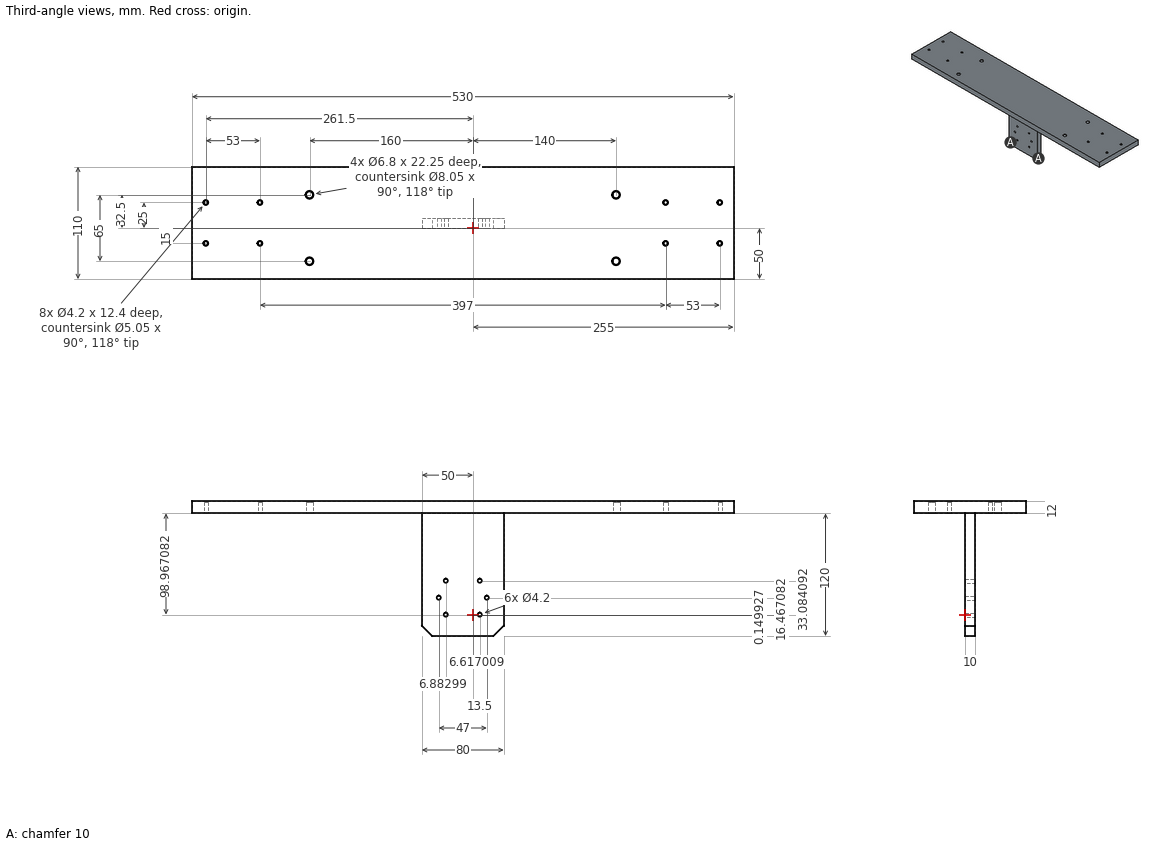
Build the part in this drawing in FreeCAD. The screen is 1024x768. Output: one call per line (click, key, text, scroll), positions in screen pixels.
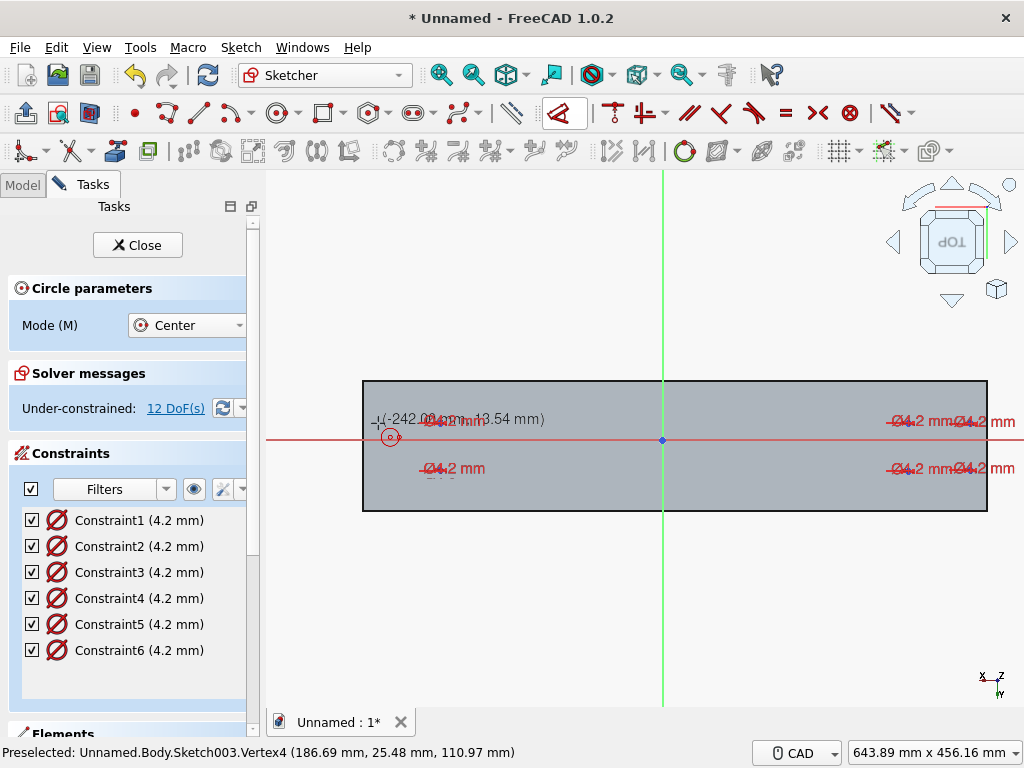
click(379, 423)
move(380, 421)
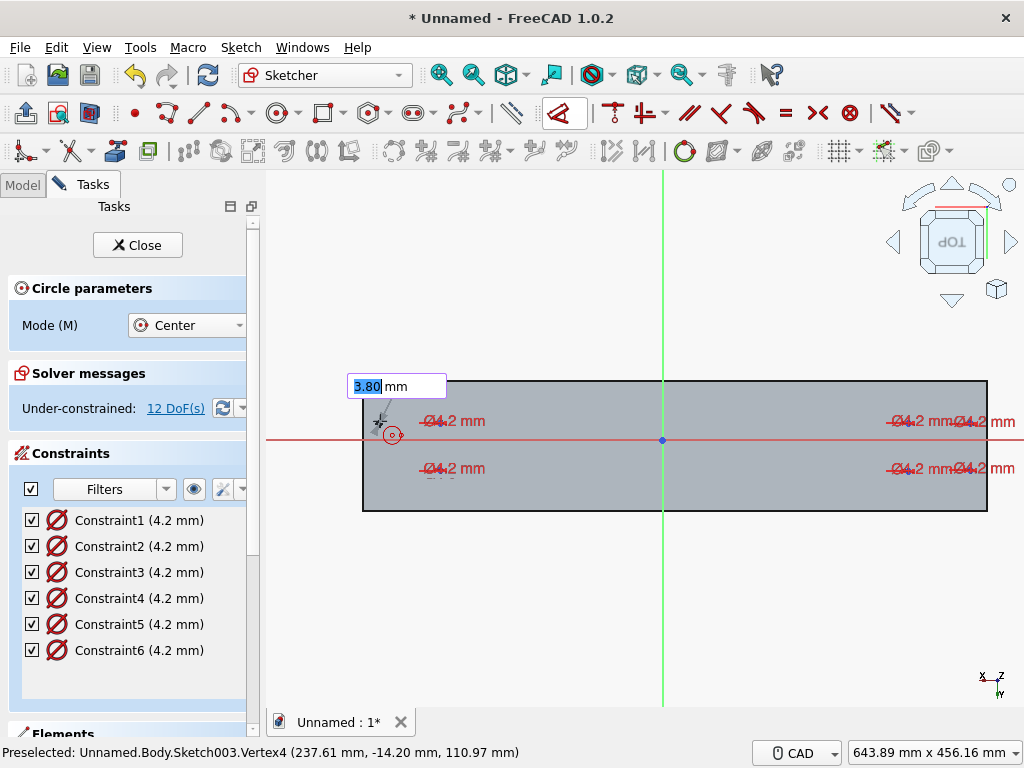
text(4.2)
key(Return)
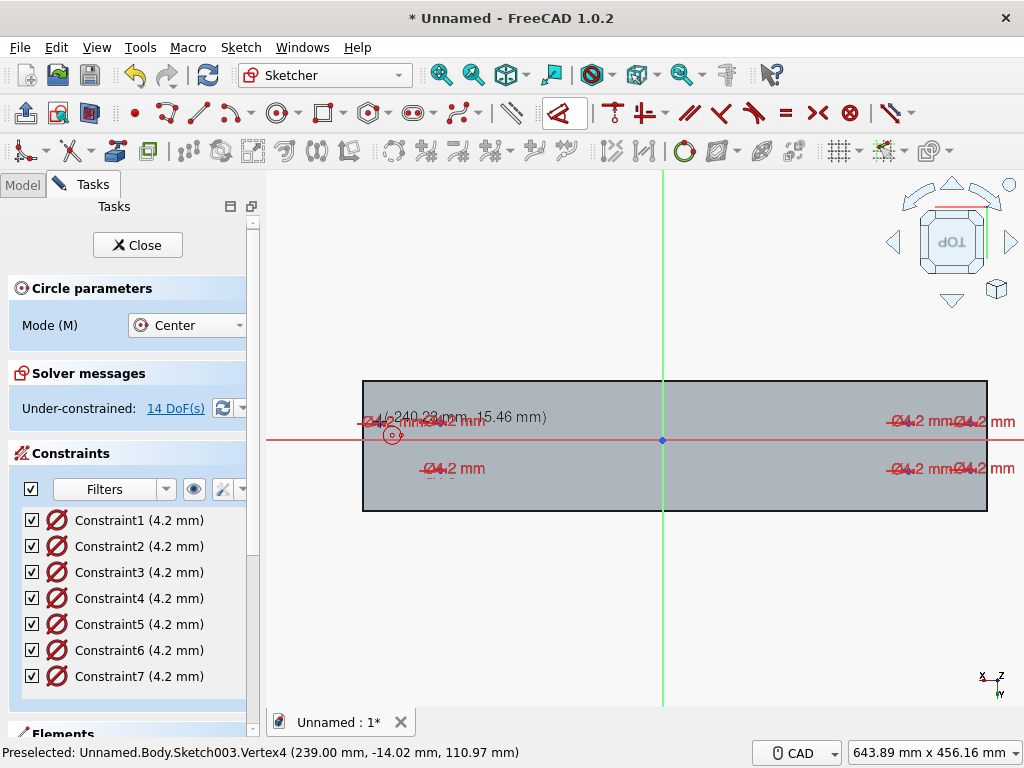
scroll(379, 470, up, 12)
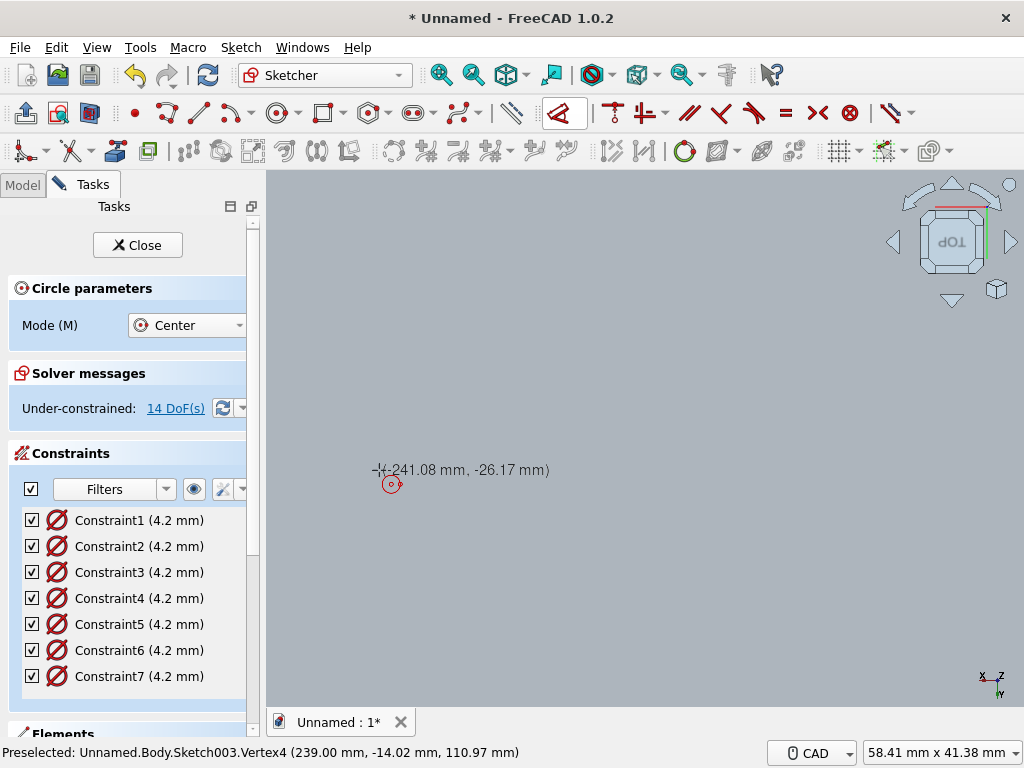
scroll(378, 454, down, 14)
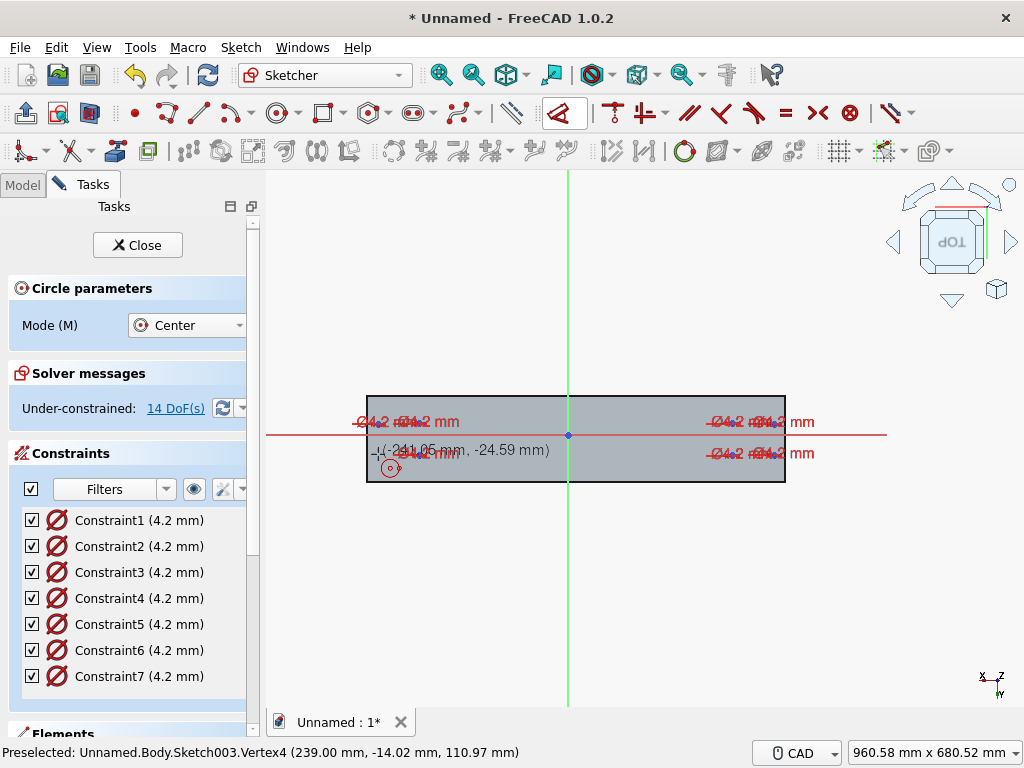
click(378, 455)
move(379, 454)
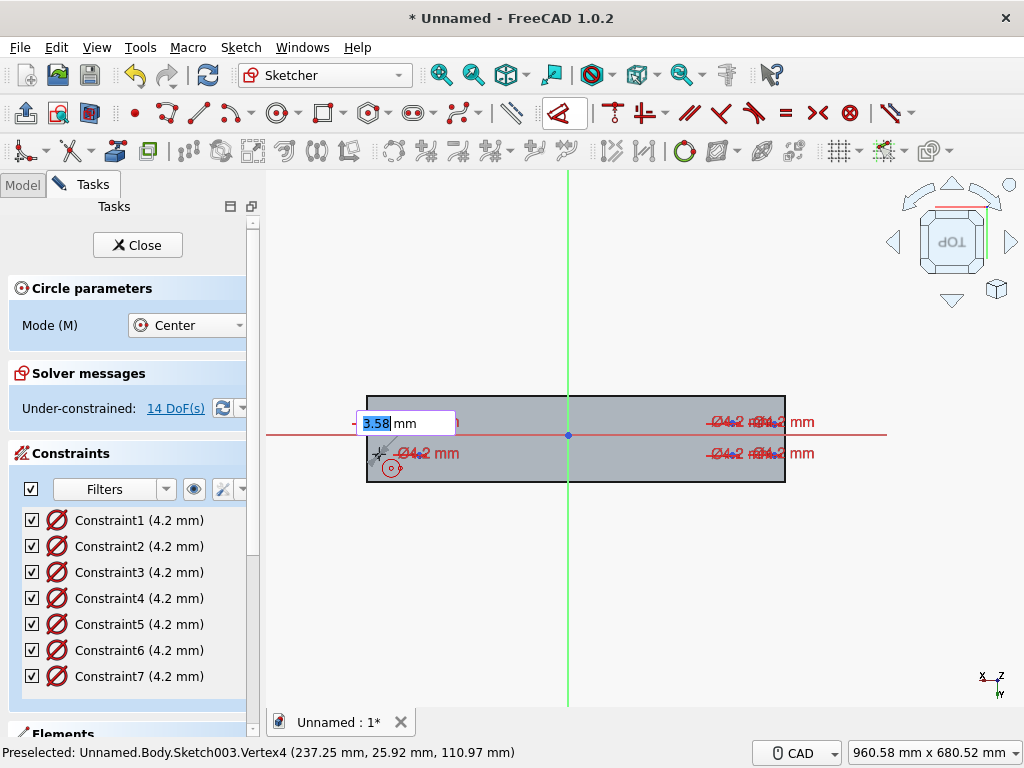
text(4.2)
key(Return)
key(Escape)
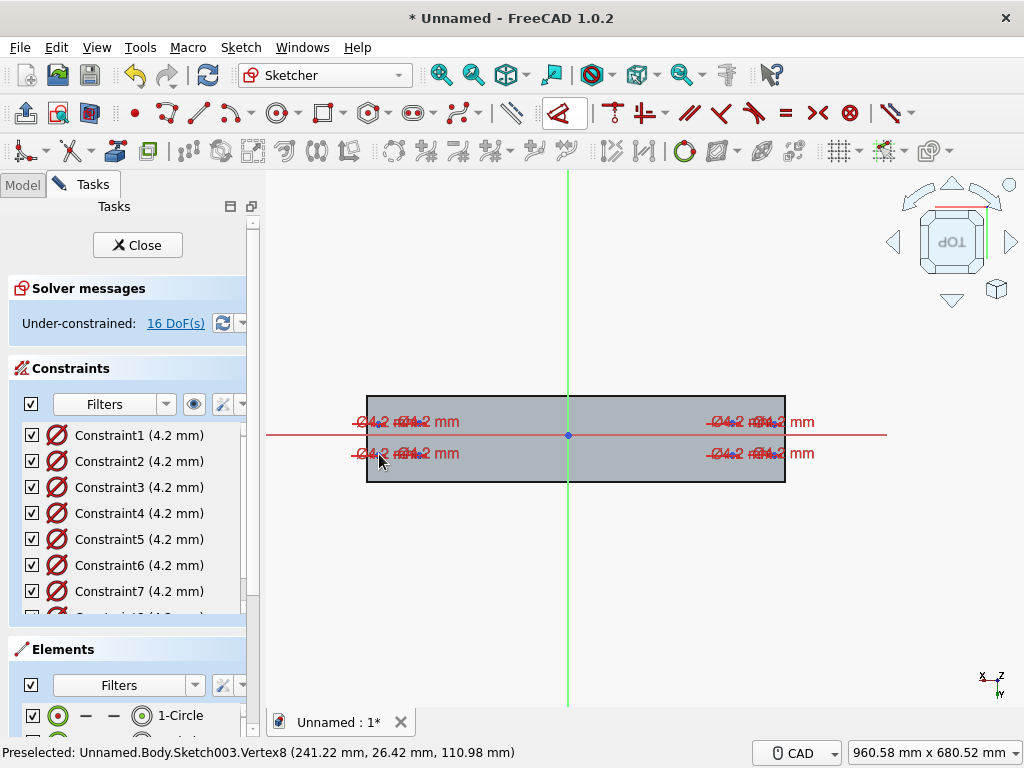
click(775, 455)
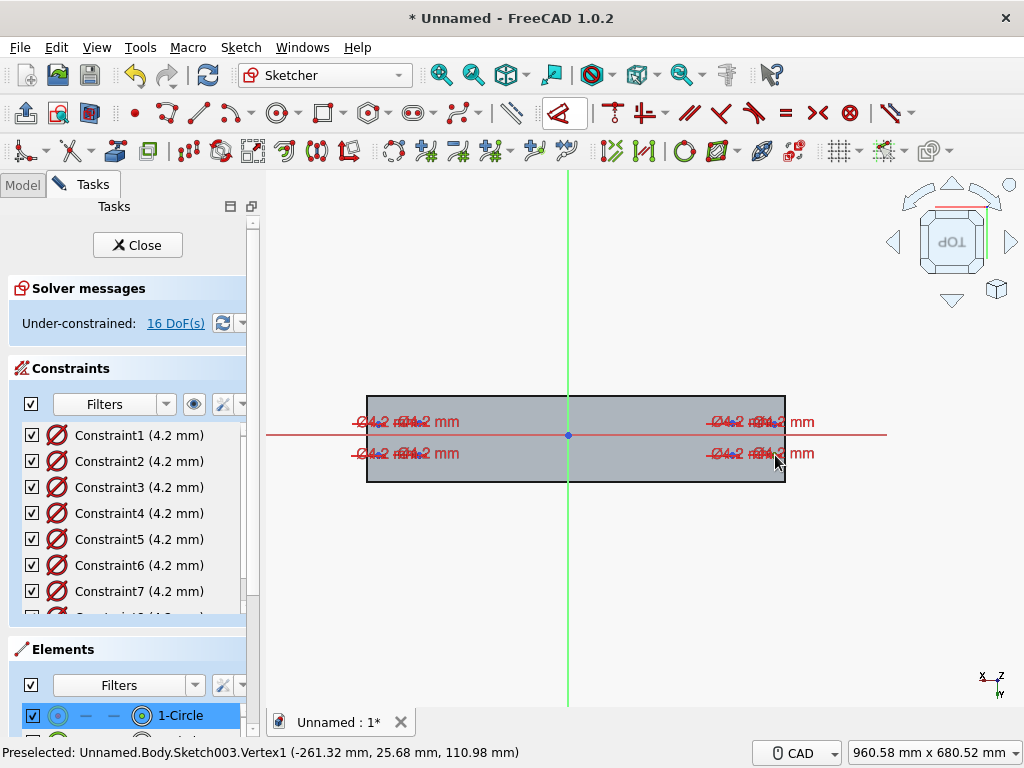
click(775, 424)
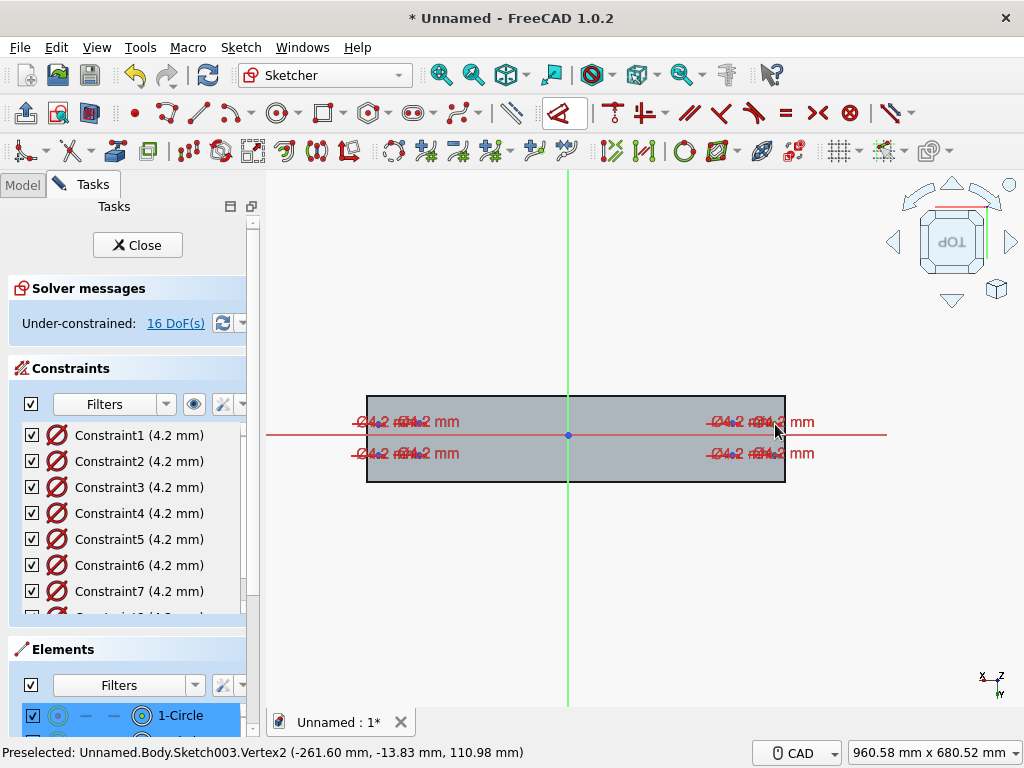
key(v)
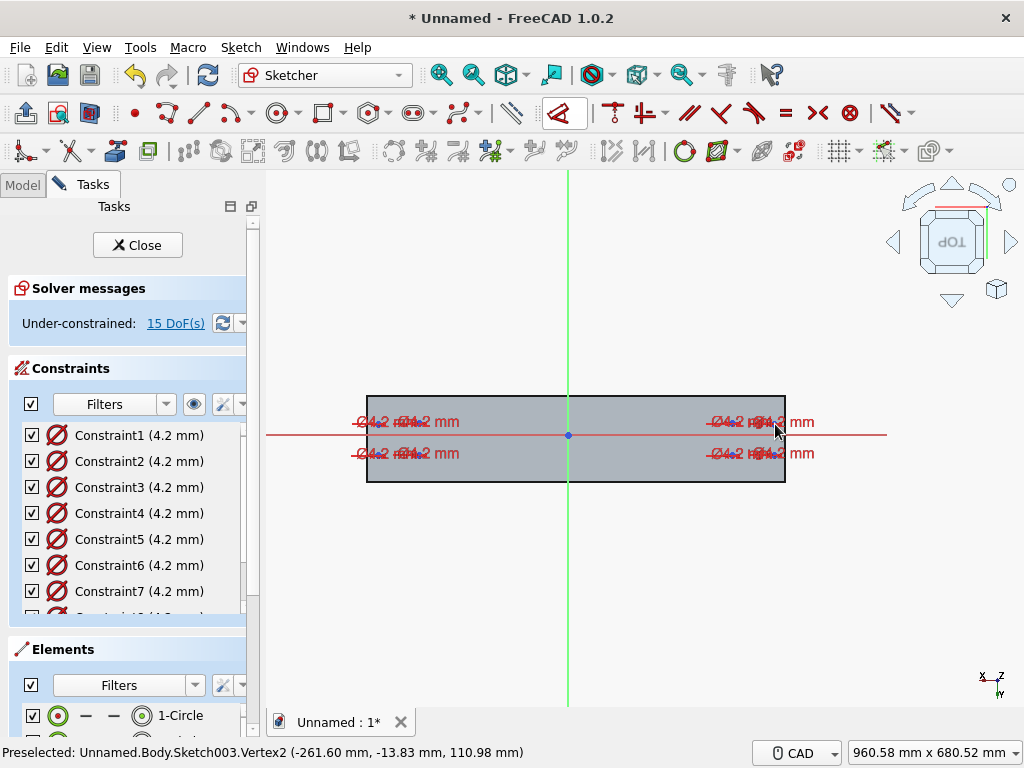
click(775, 455)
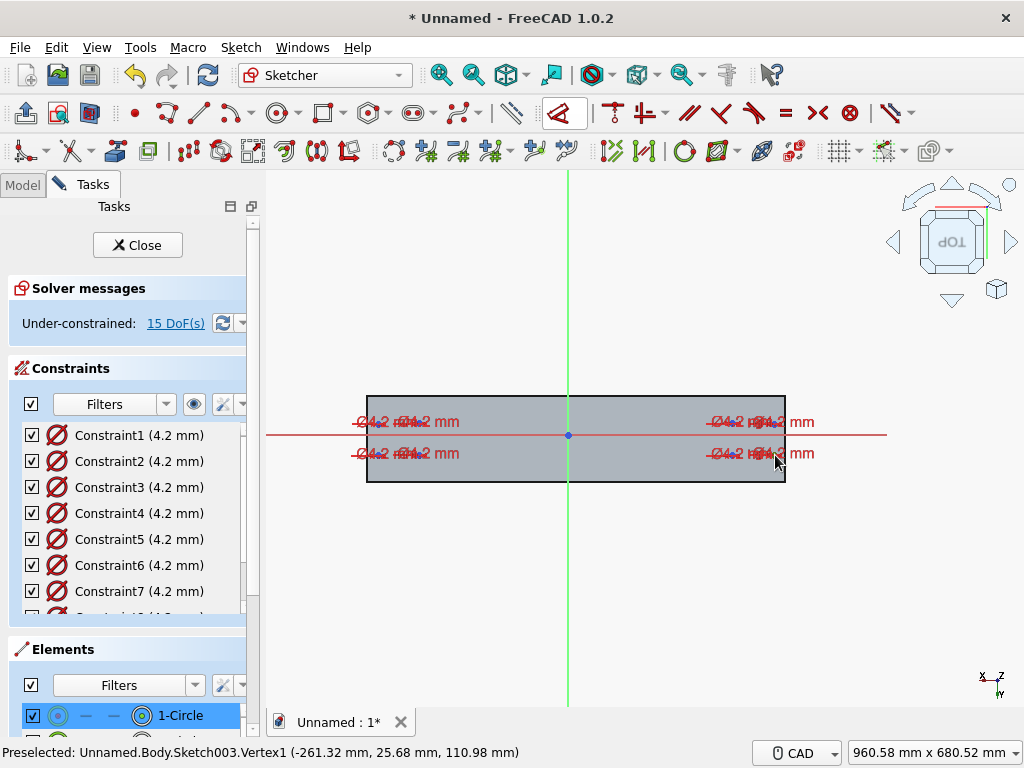
click(733, 456)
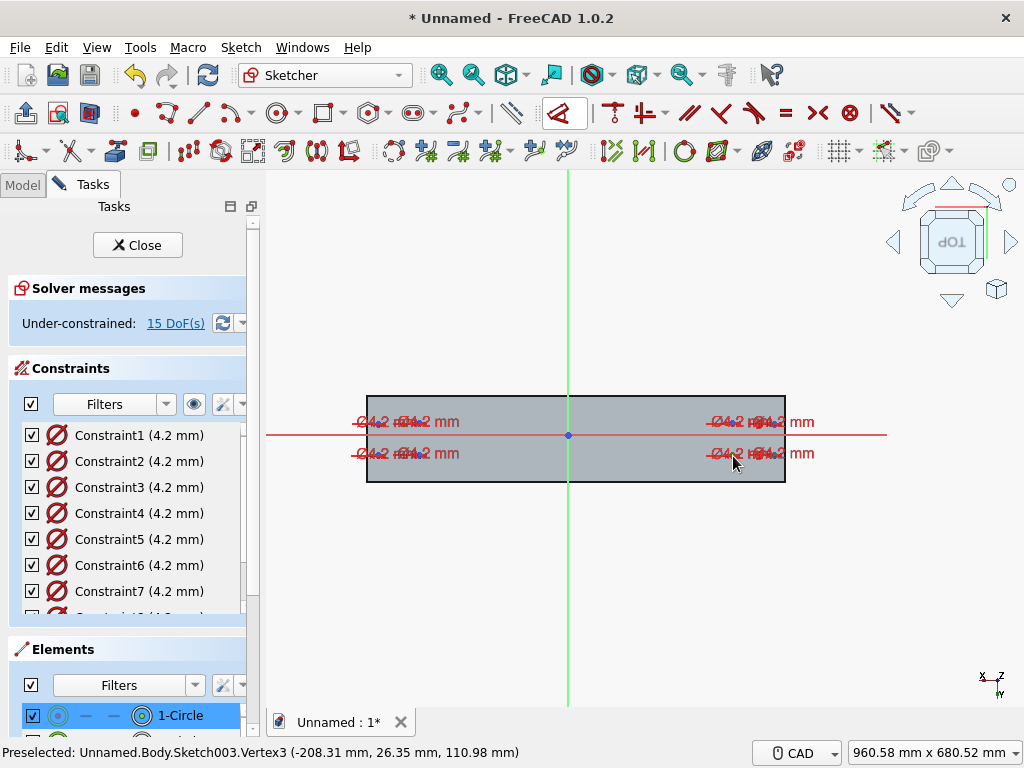
key(h)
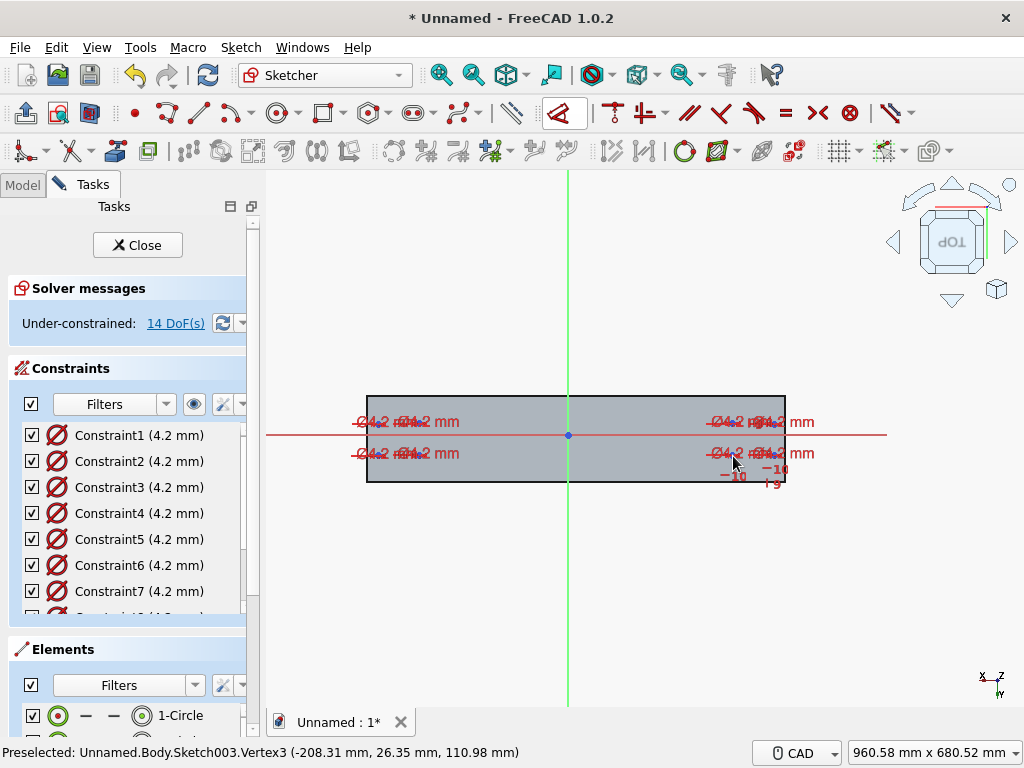
click(733, 455)